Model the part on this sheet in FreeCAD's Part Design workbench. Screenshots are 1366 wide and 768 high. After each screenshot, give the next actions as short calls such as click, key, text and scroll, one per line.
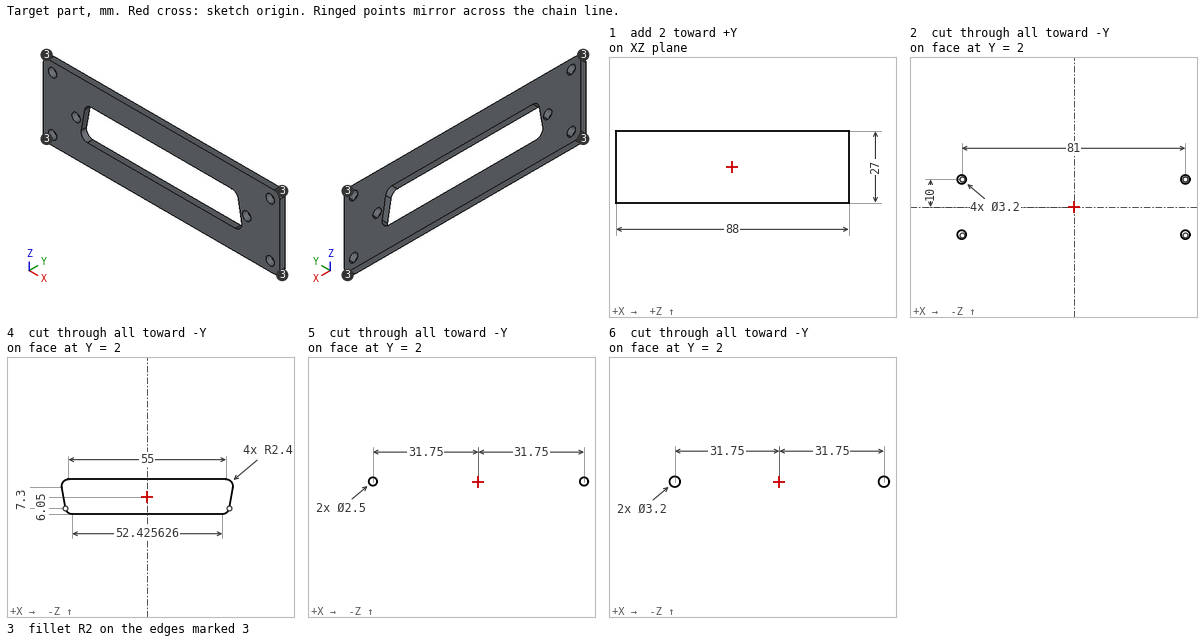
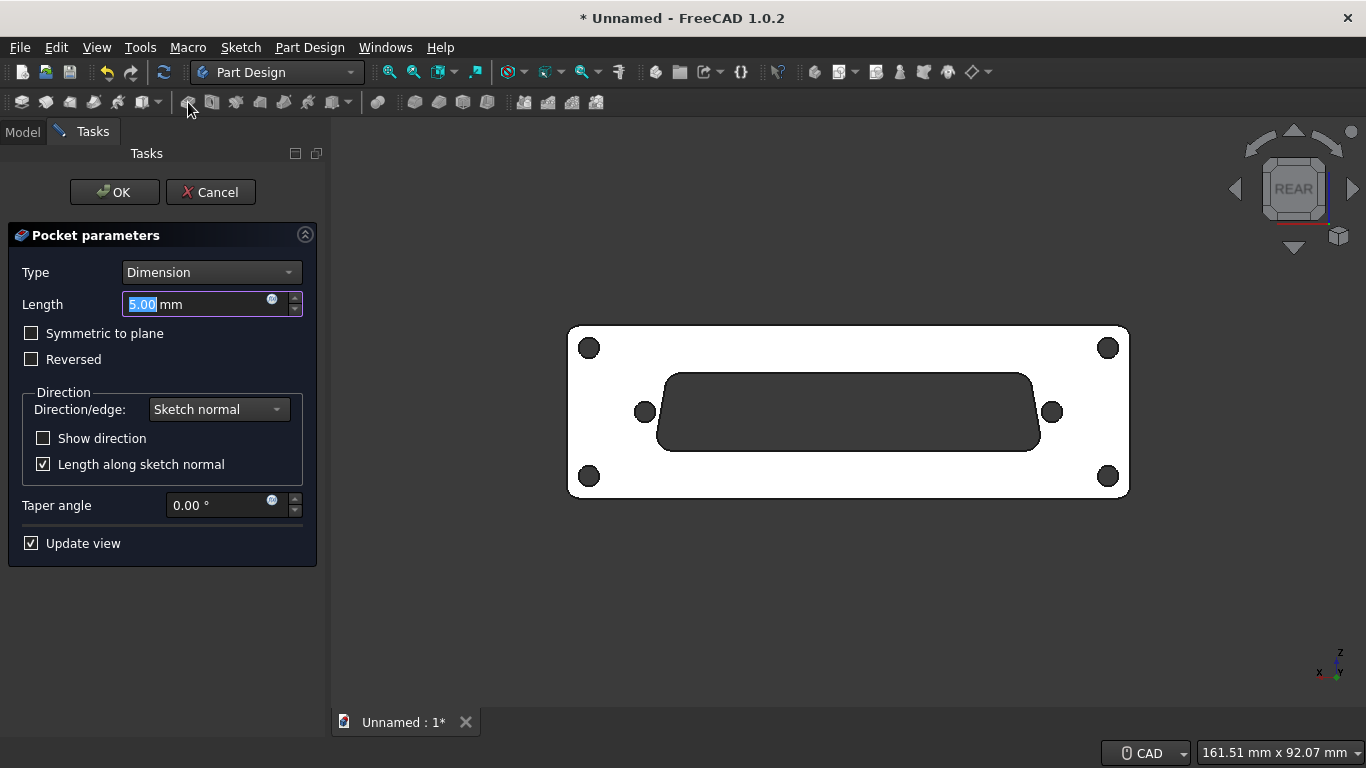
click(212, 272)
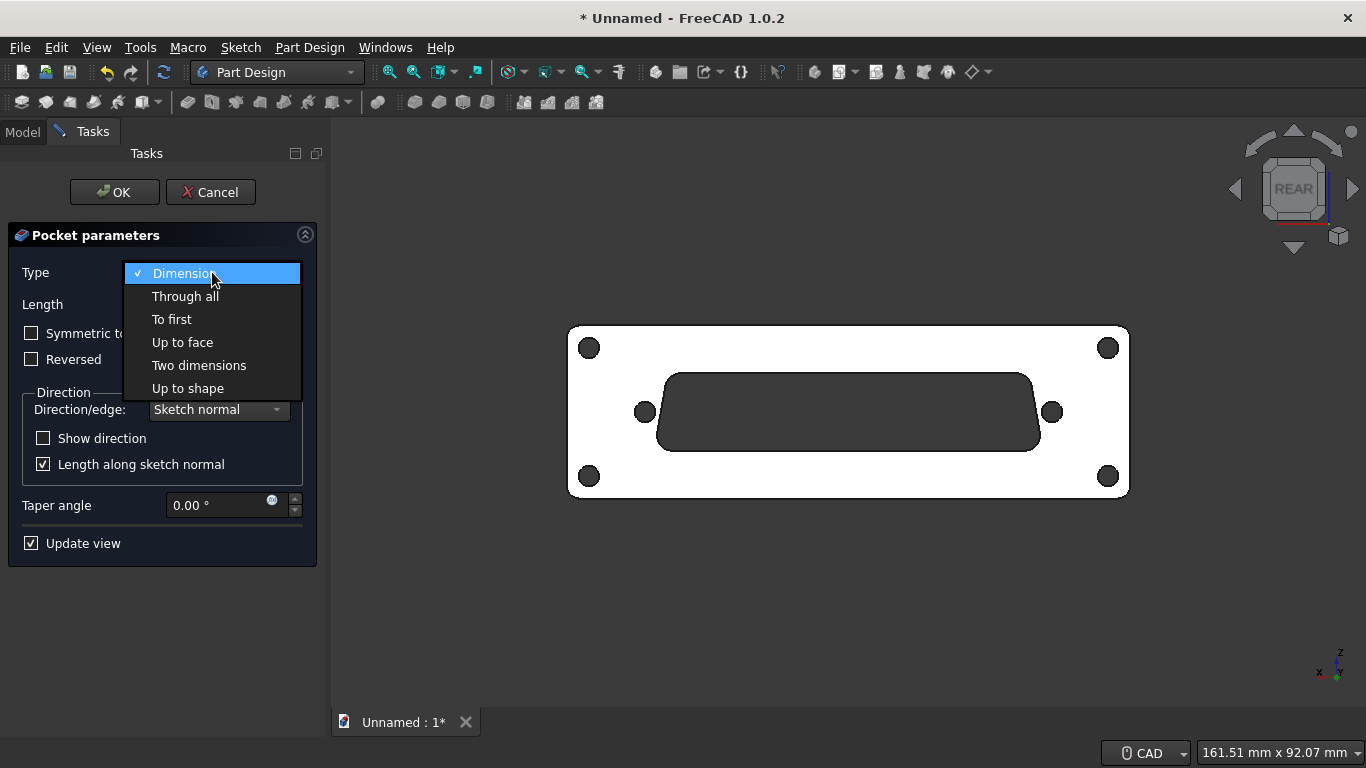
click(212, 296)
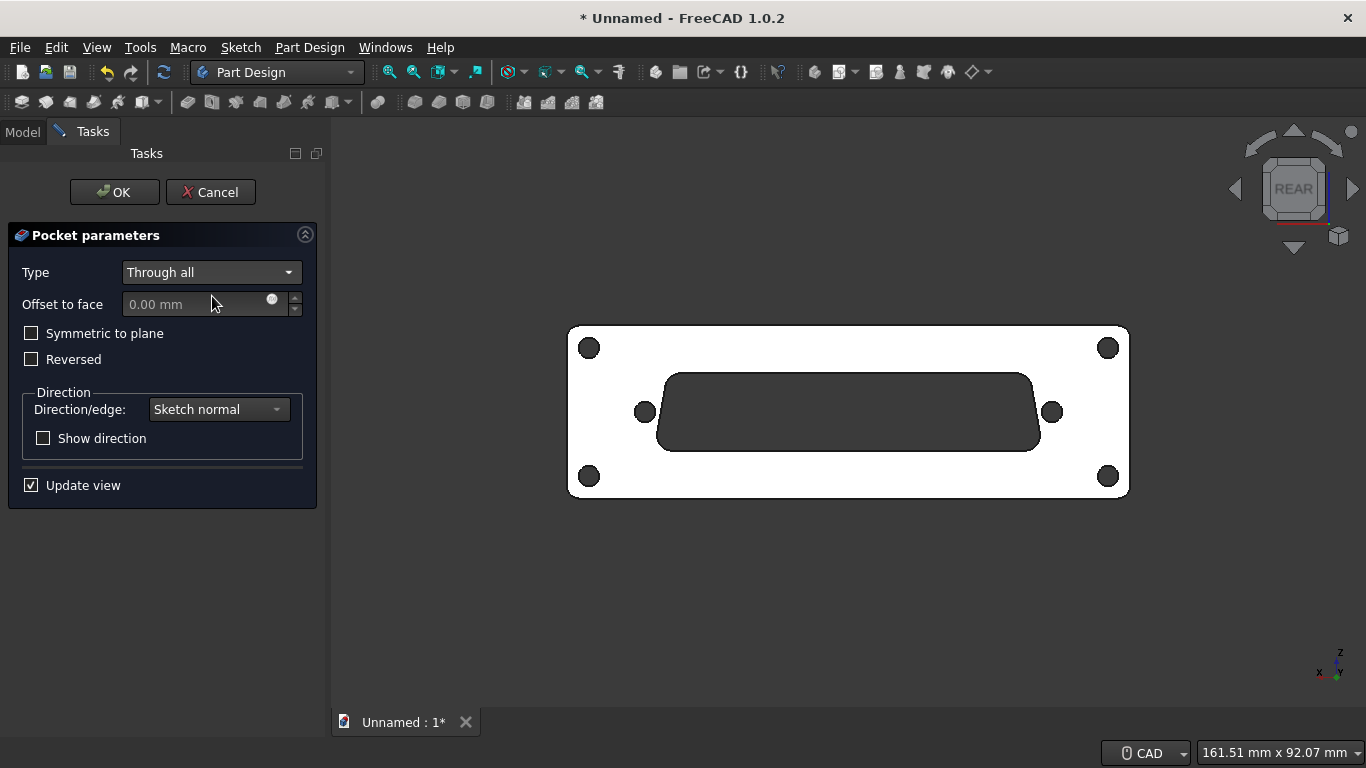
click(115, 192)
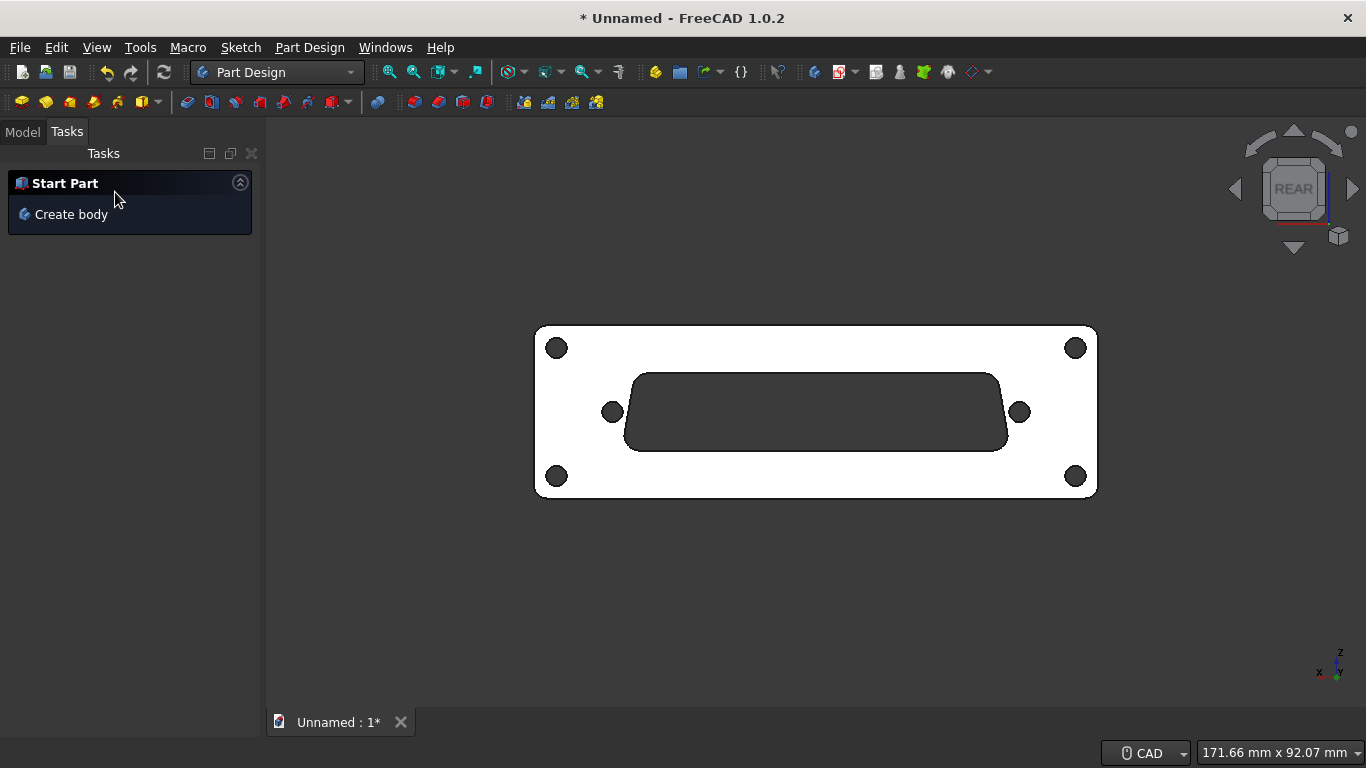
key(0)